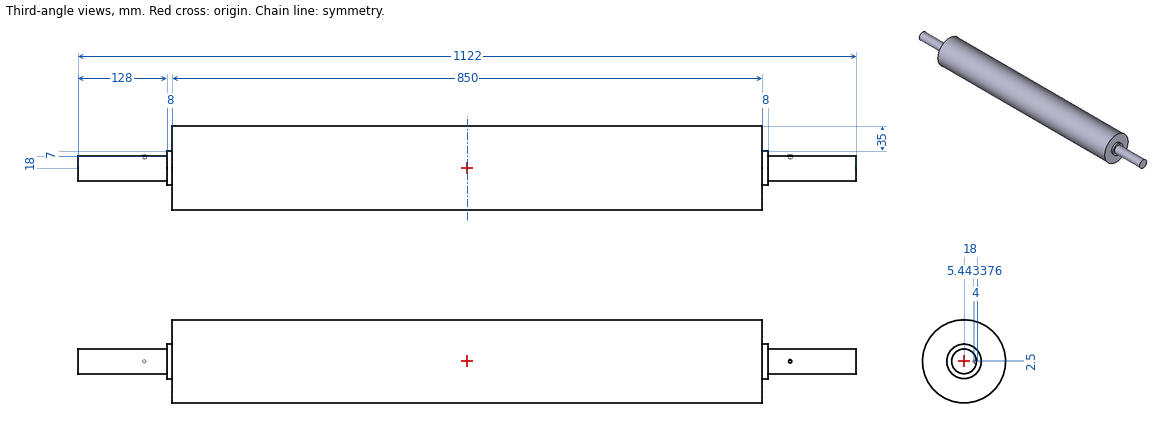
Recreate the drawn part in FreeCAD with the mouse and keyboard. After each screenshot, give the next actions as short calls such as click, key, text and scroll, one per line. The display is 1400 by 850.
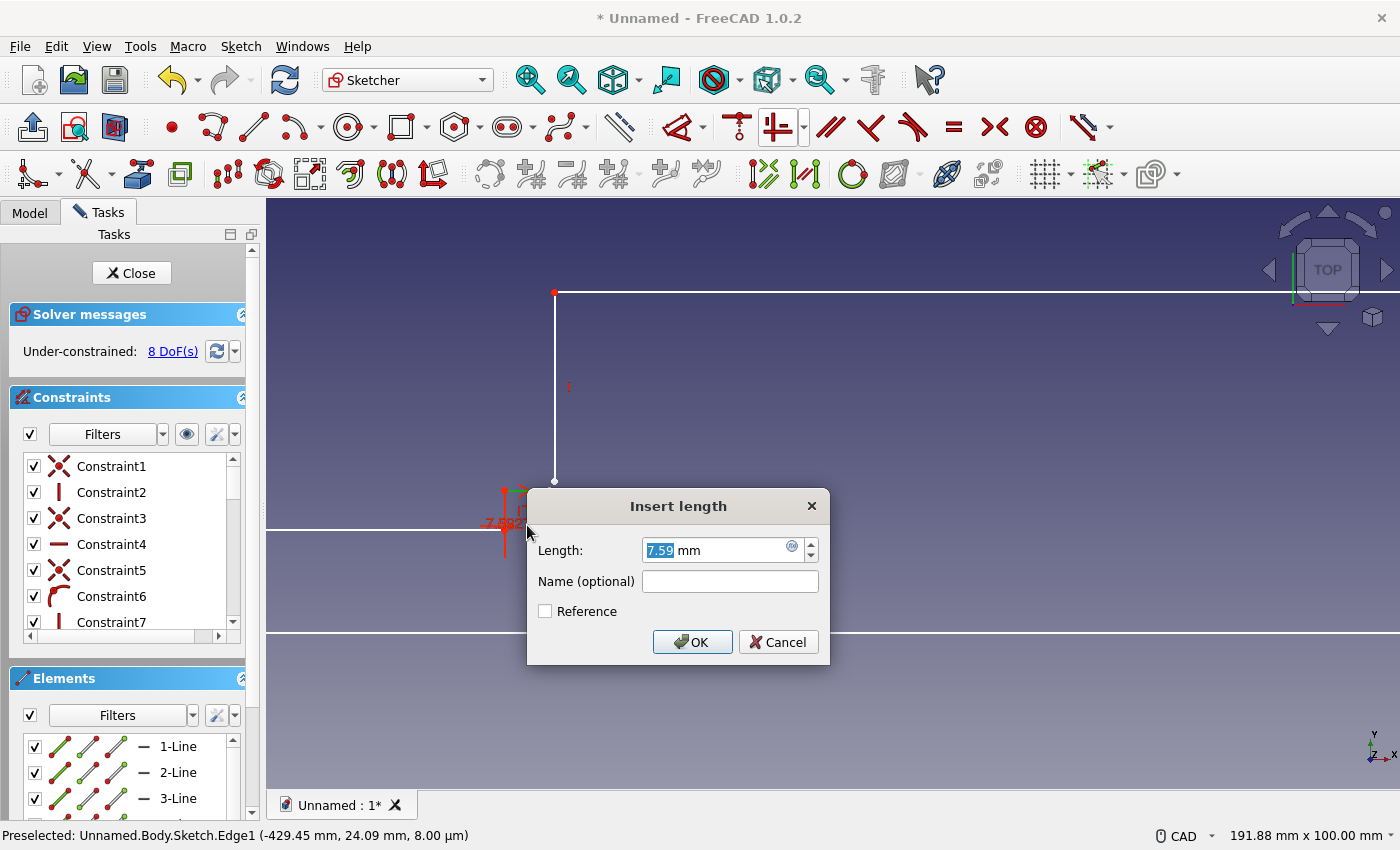
text(8)
key(Return)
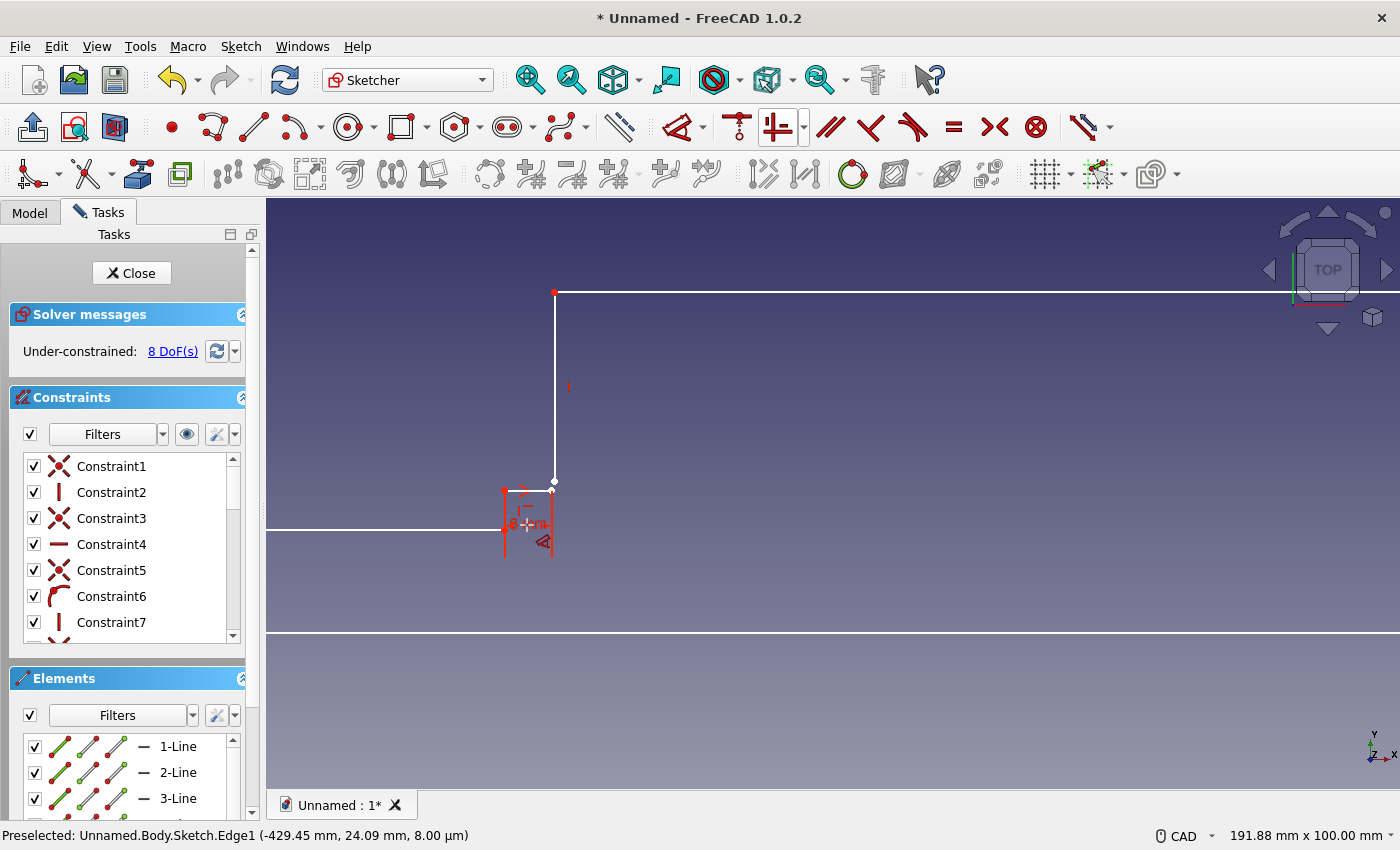
click(505, 503)
click(471, 502)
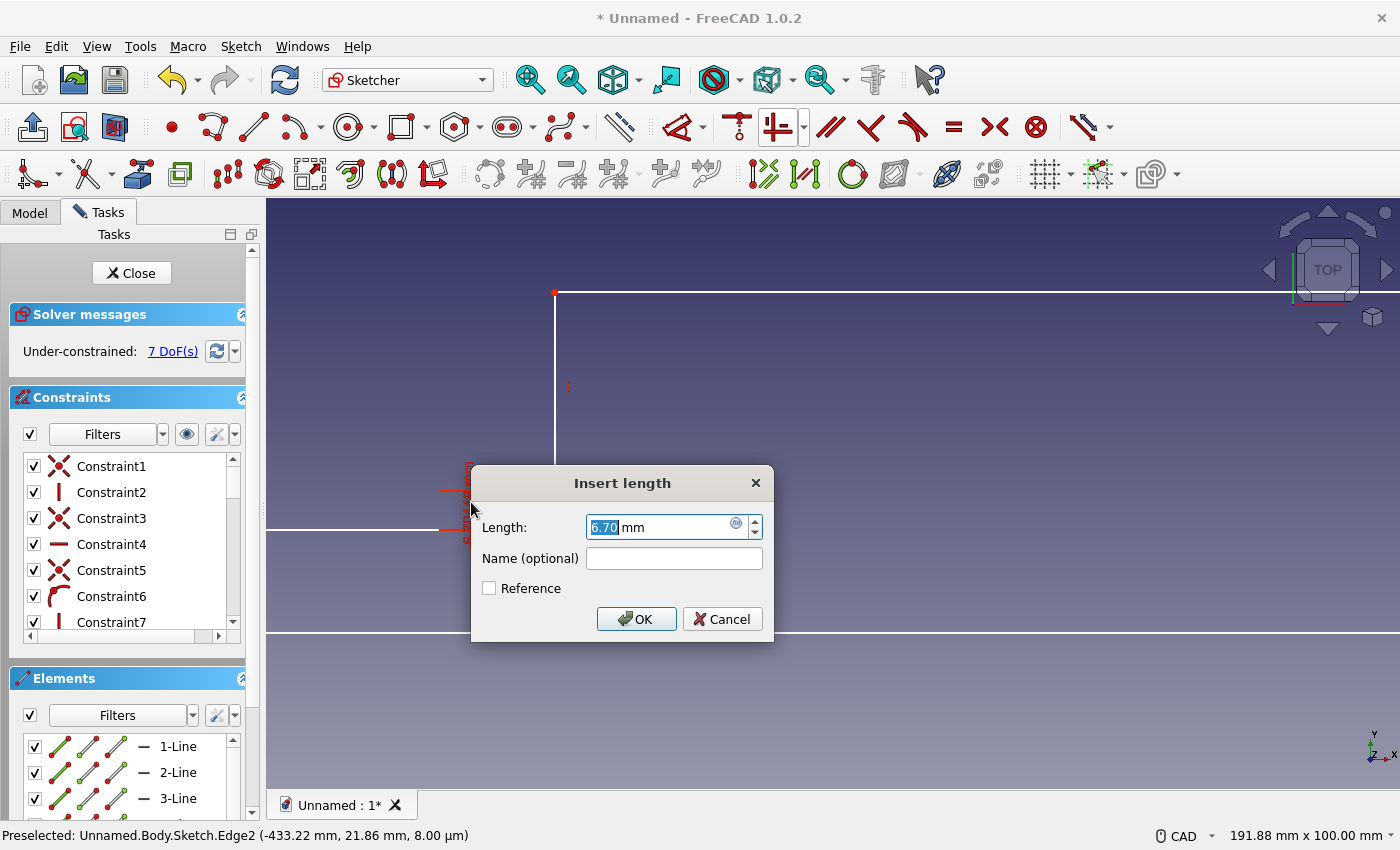
text(7)
key(Return)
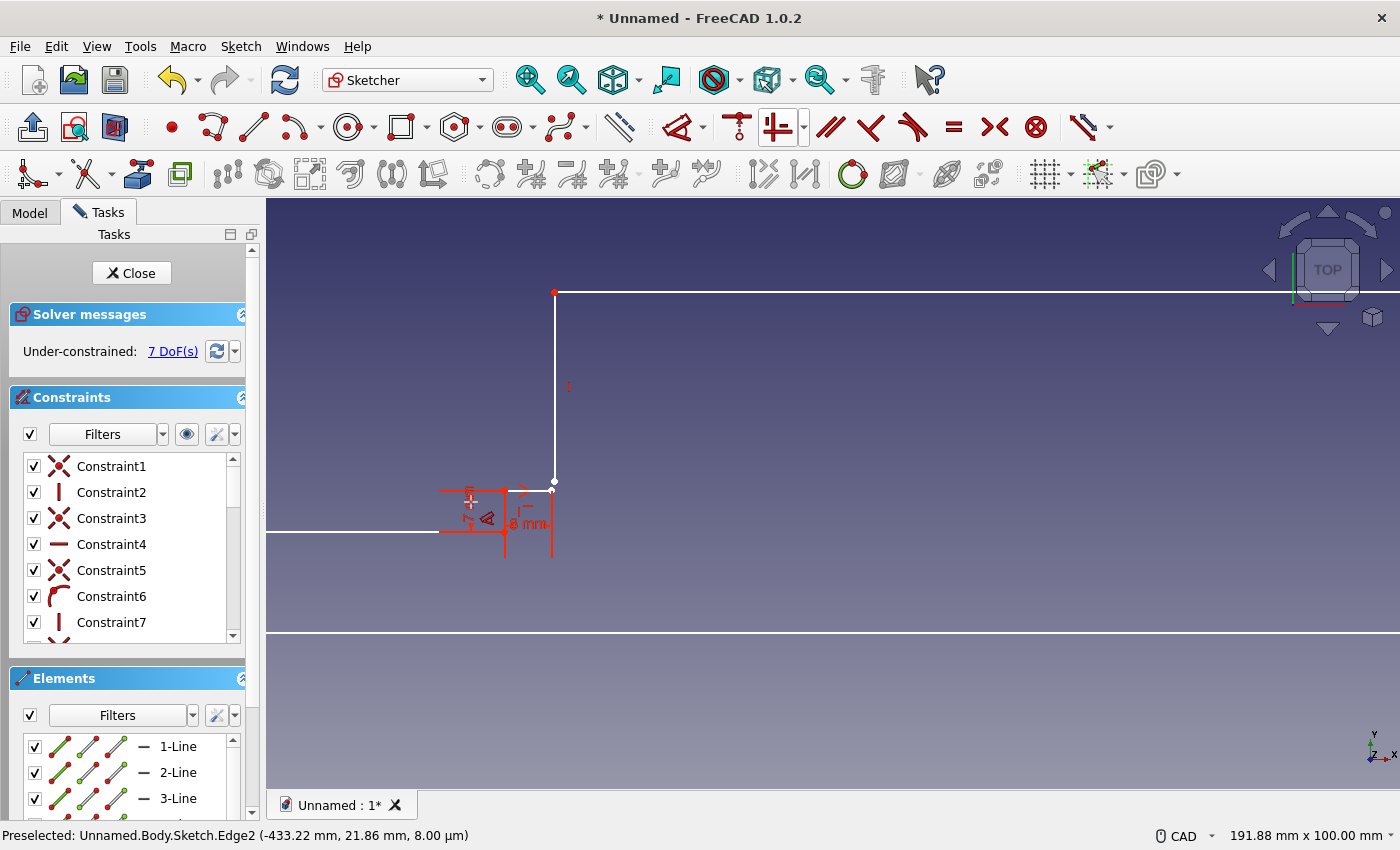
scroll(535, 497, down, 12)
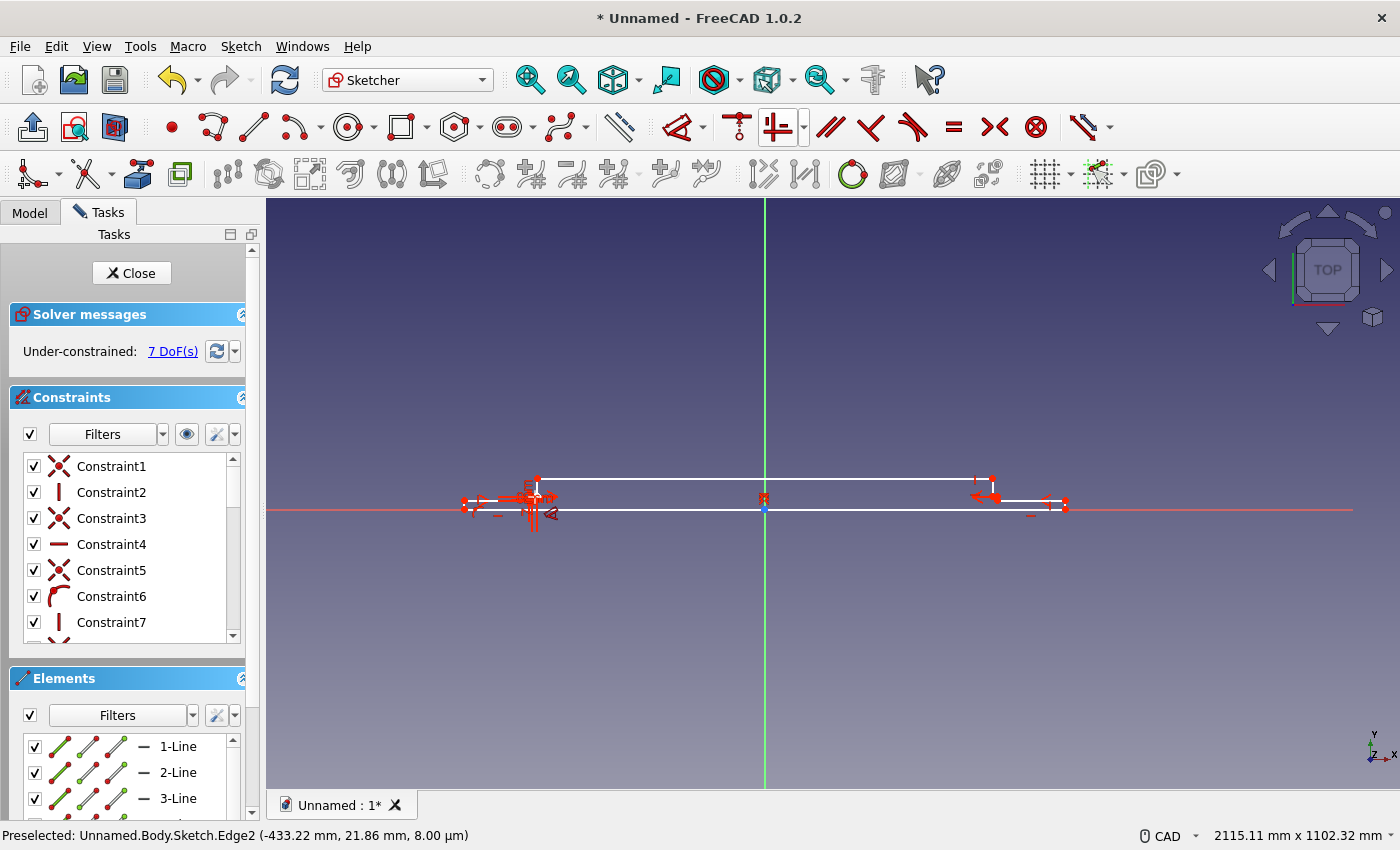
scroll(996, 497, up, 12)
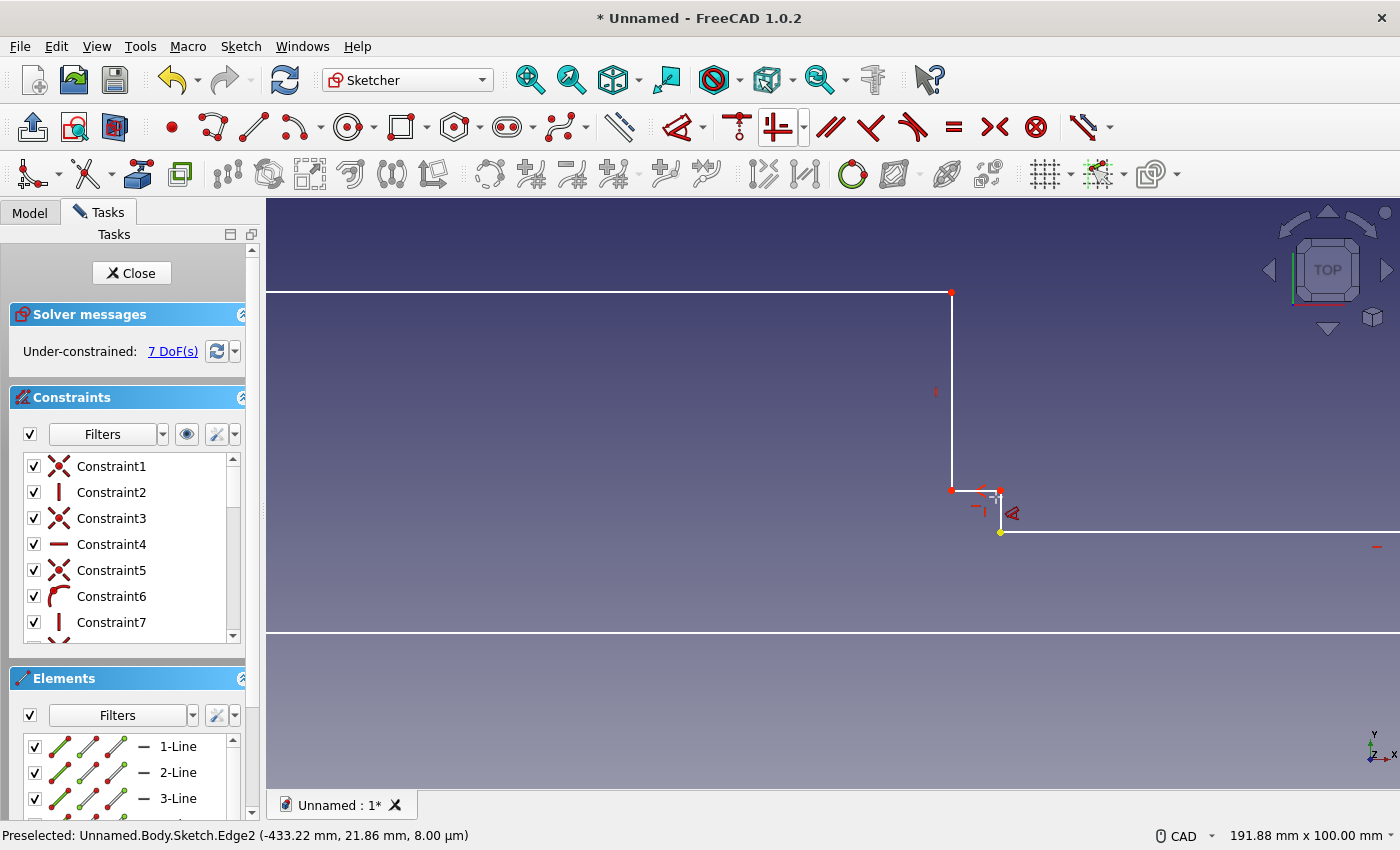
click(986, 491)
click(976, 525)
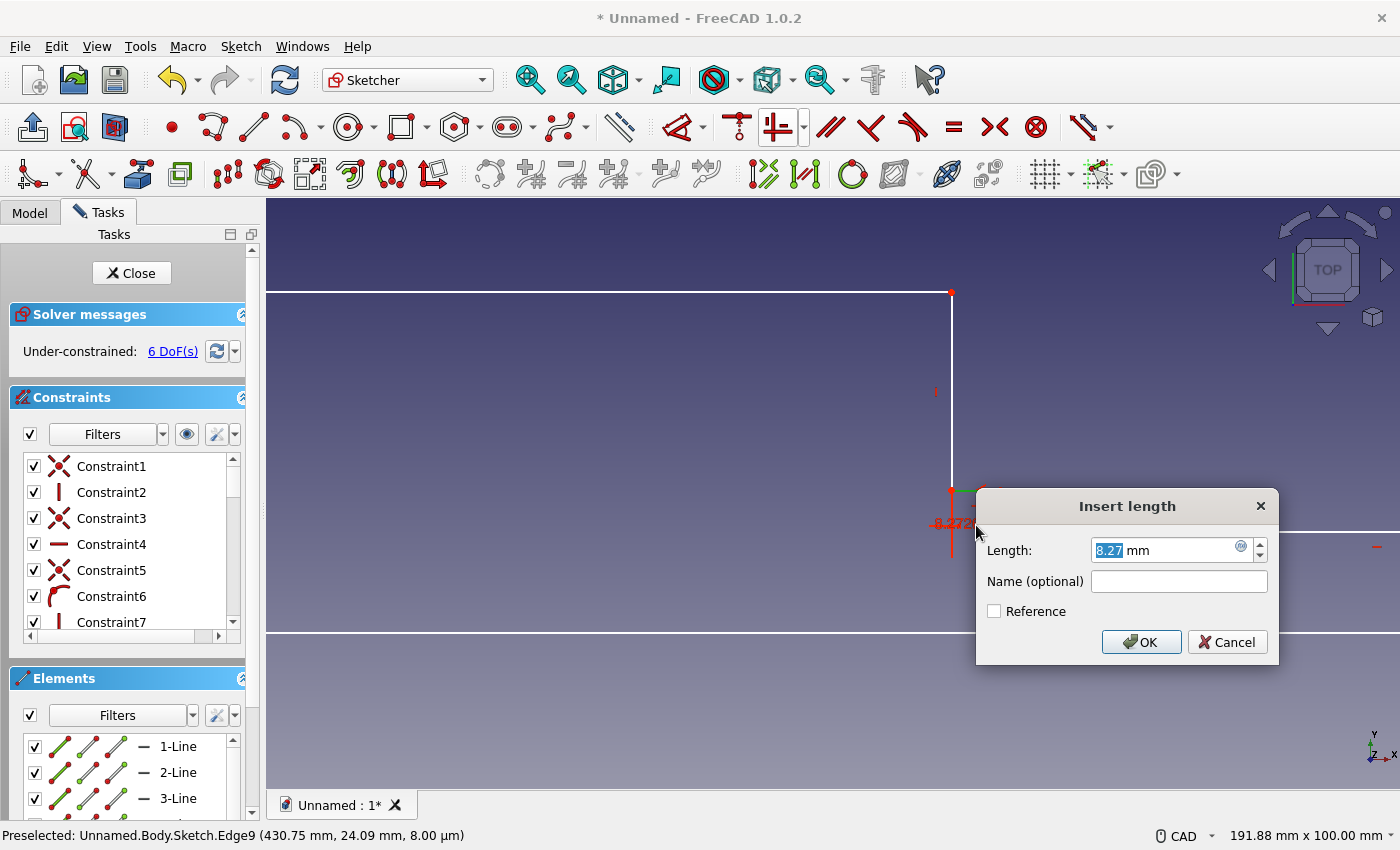
text(8)
key(Return)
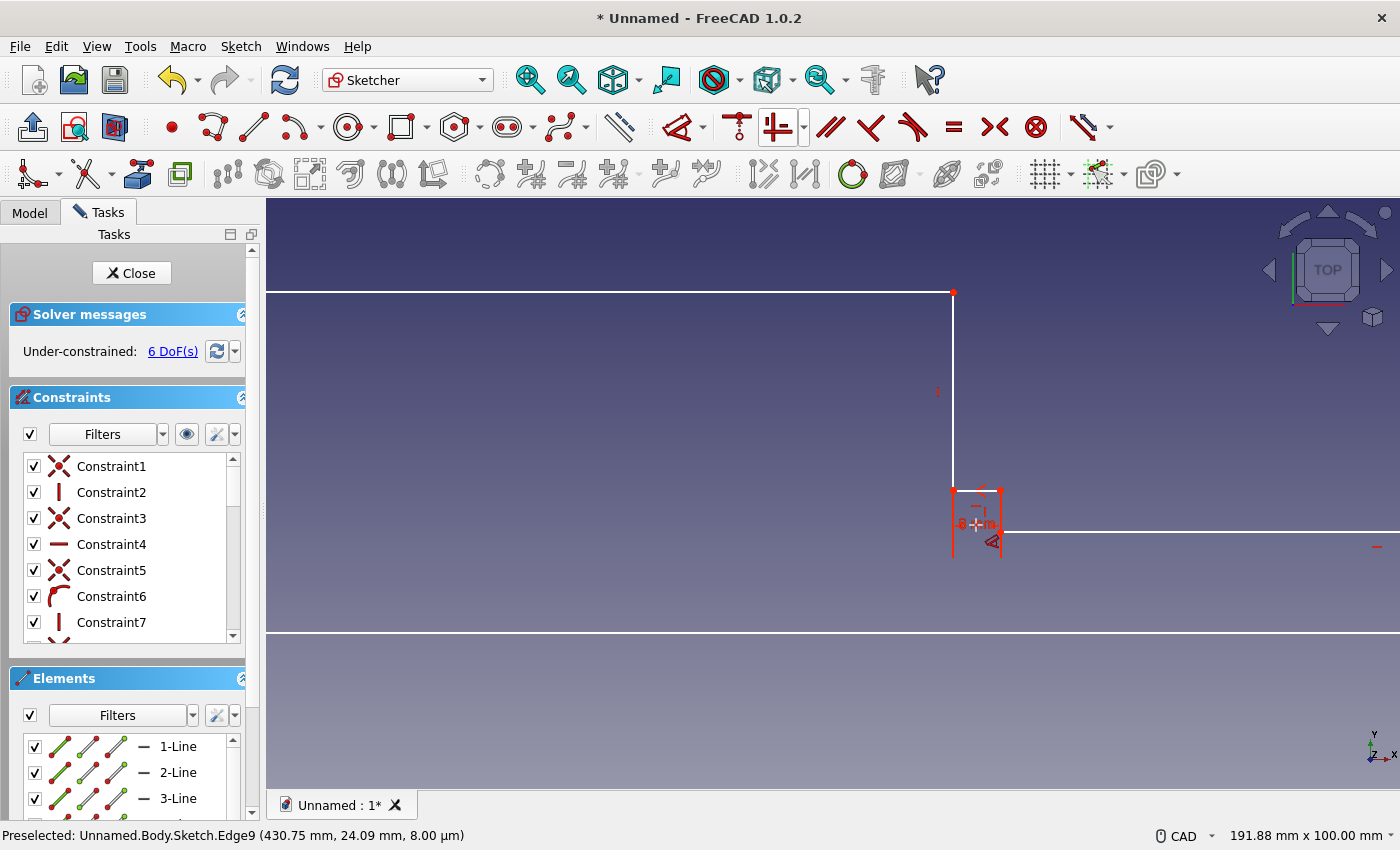
scroll(996, 497, down, 12)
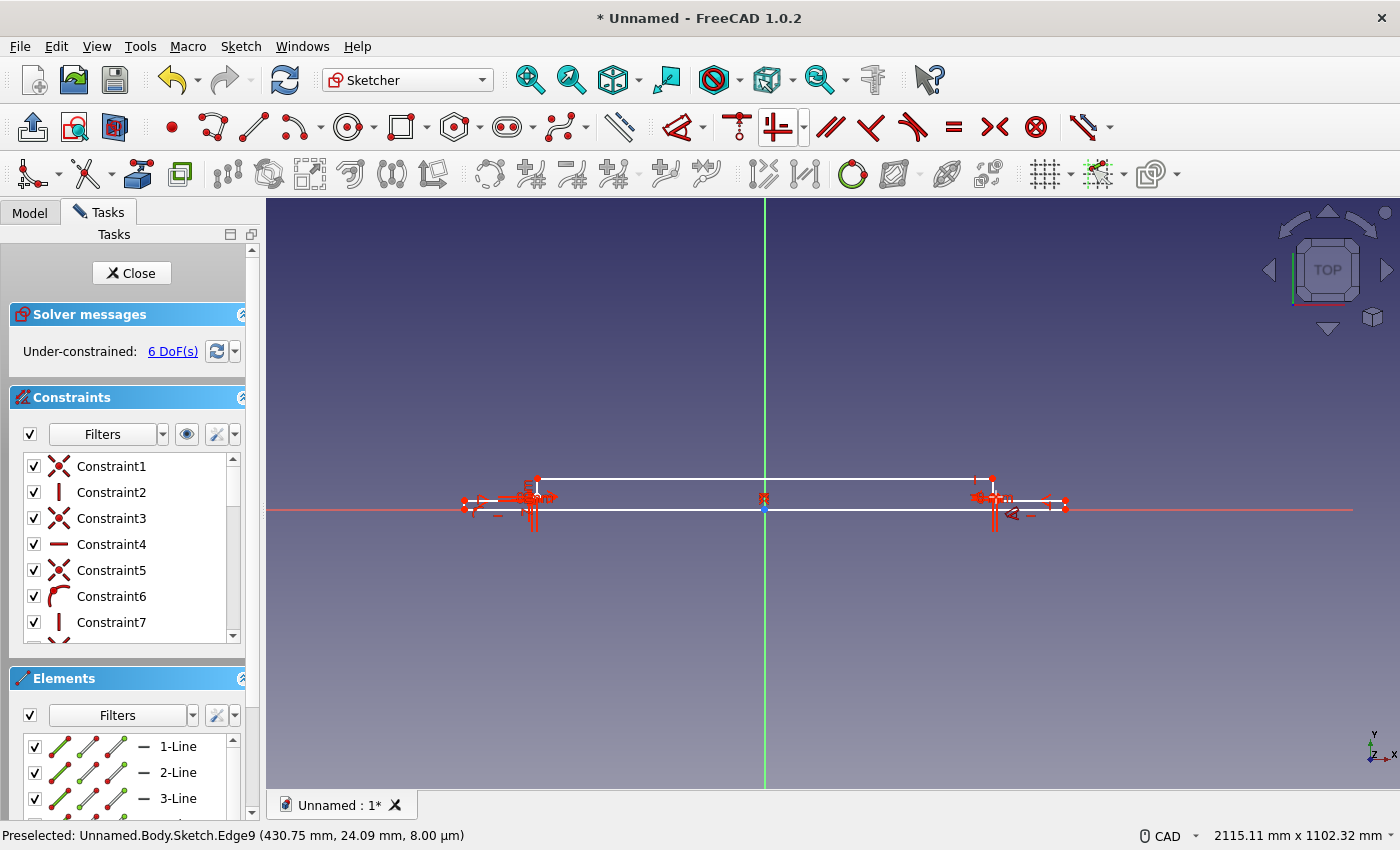
scroll(464, 503, up, 9)